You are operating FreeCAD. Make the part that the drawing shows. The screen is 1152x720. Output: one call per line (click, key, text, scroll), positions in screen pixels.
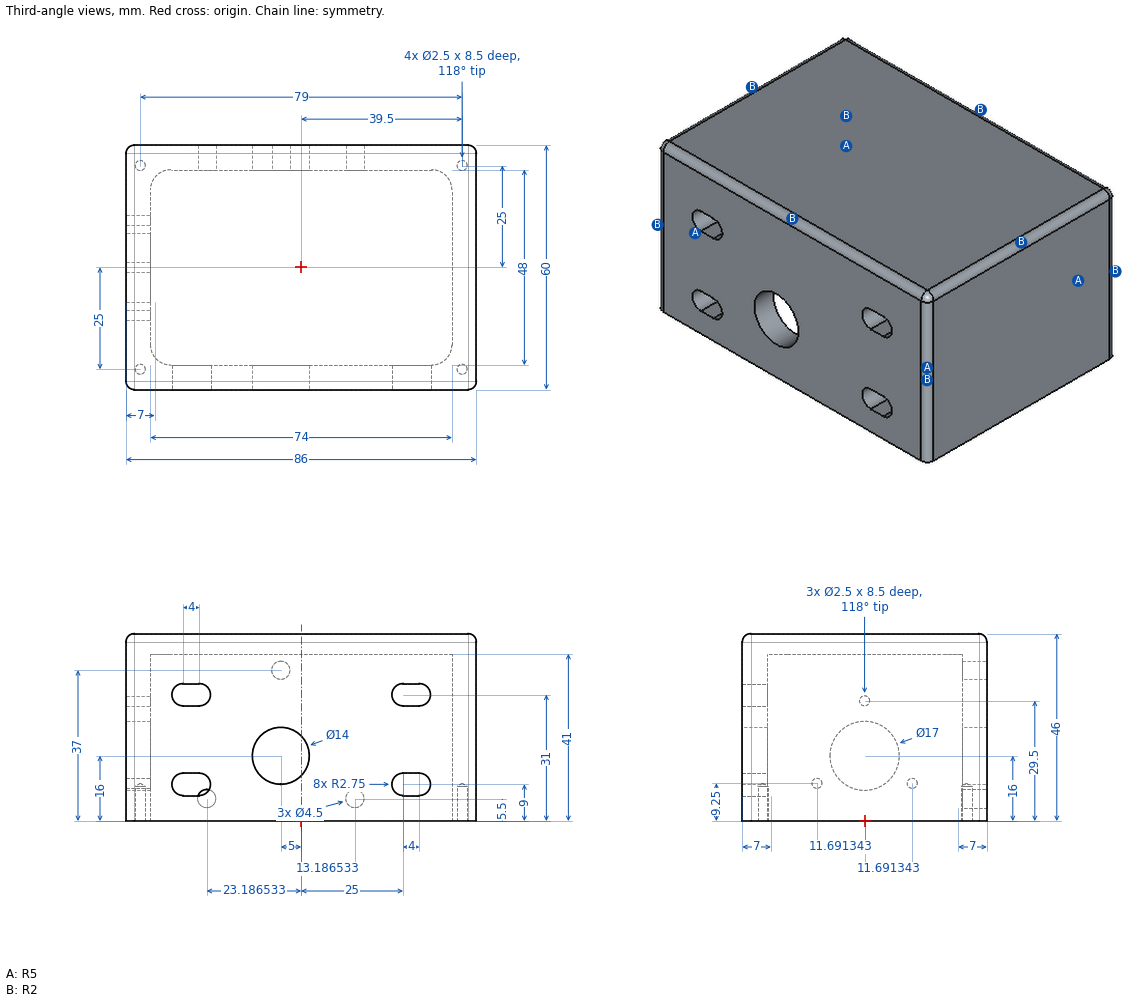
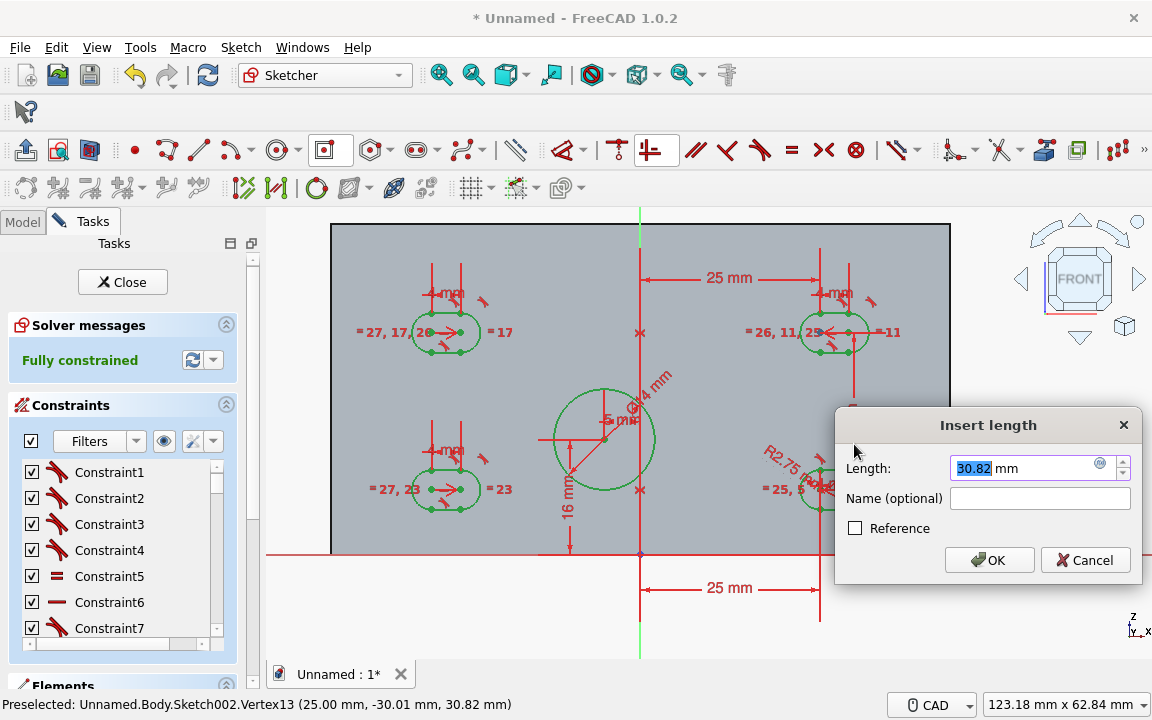
text(31)
key(Return)
key(Escape)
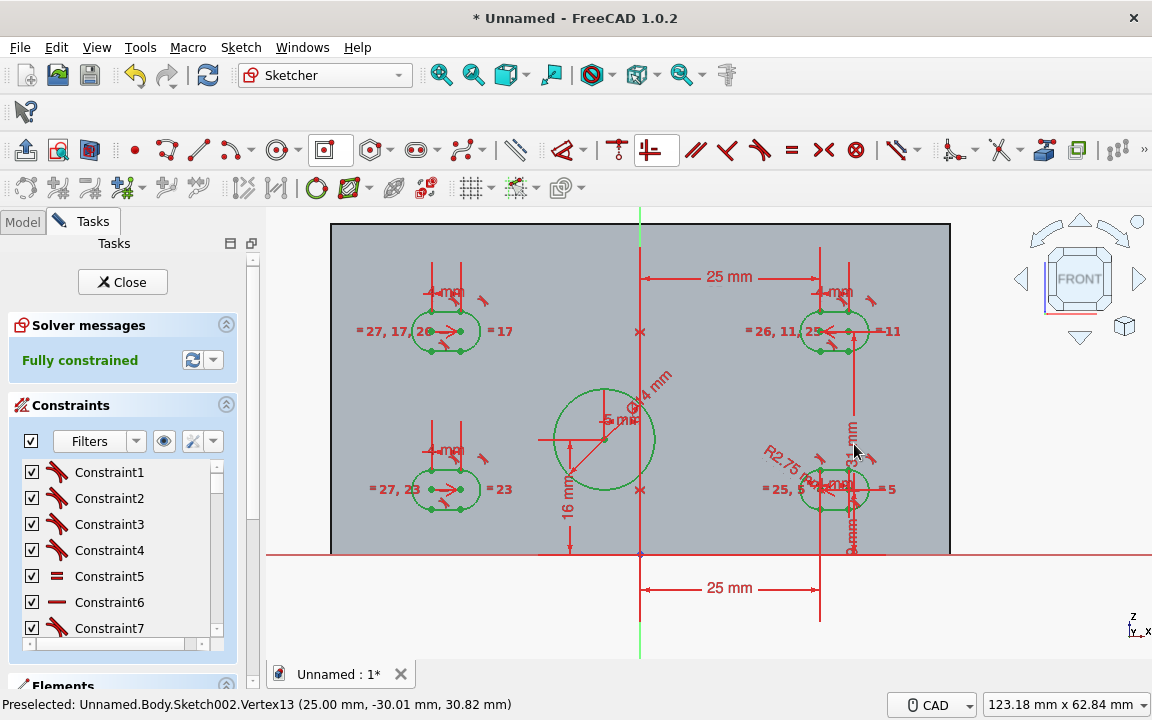
click(123, 282)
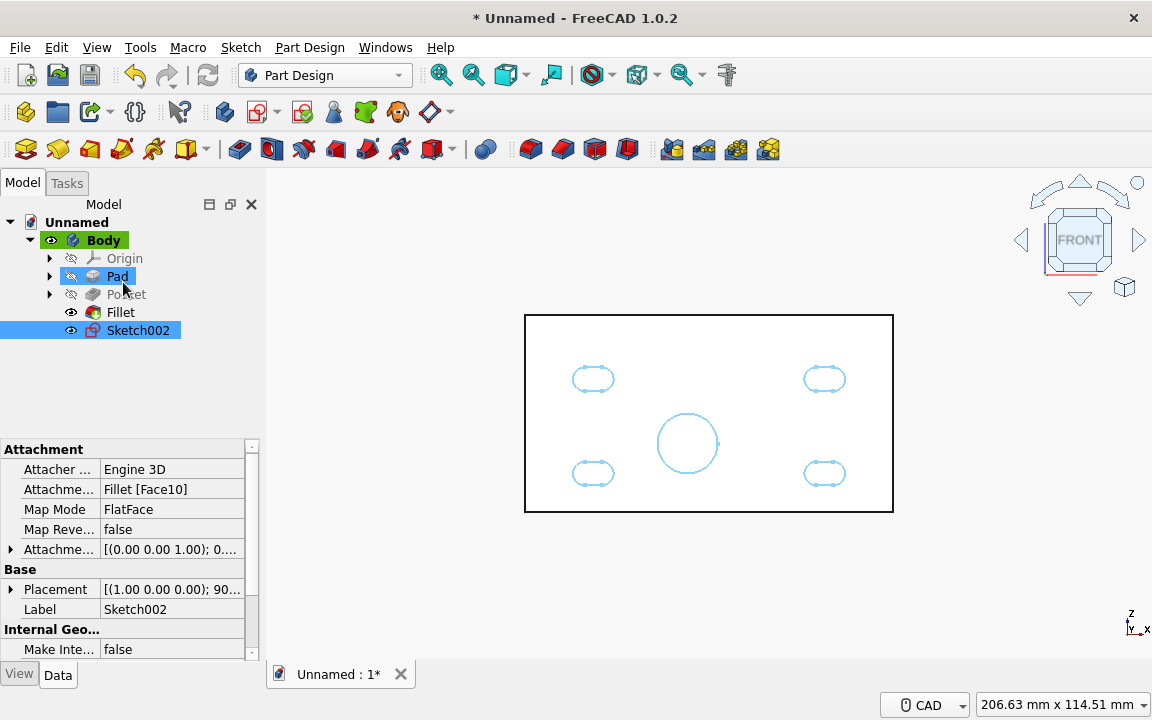
click(240, 150)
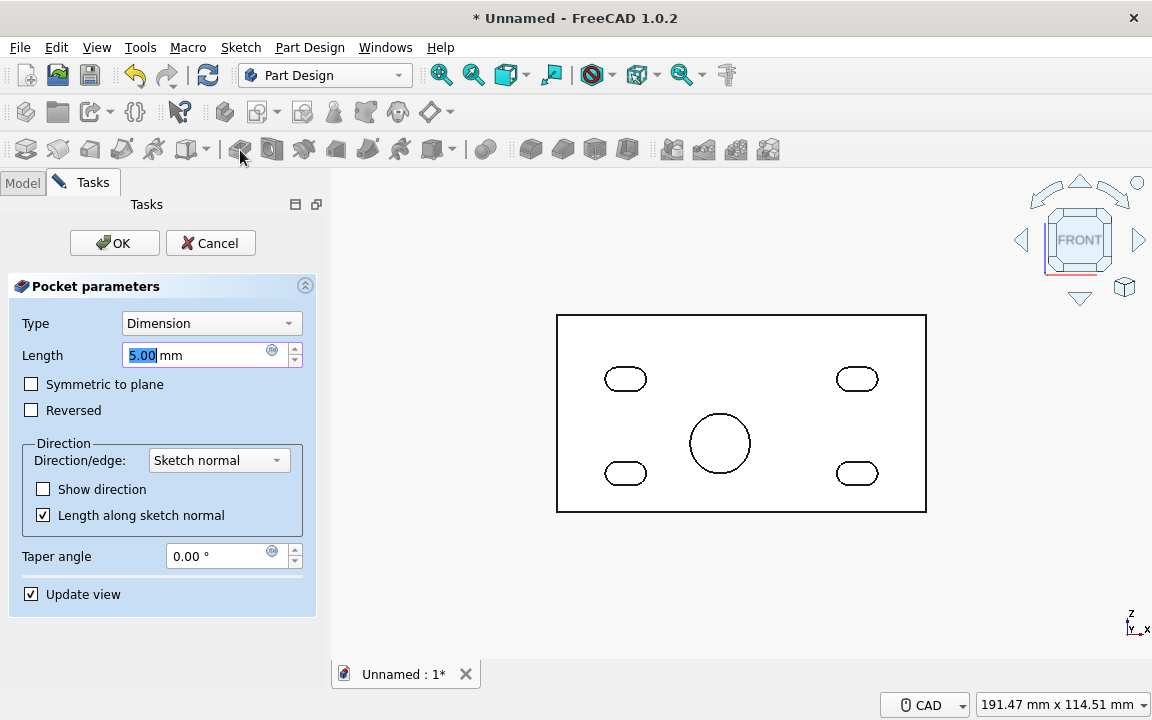
text(7)
key(Tab)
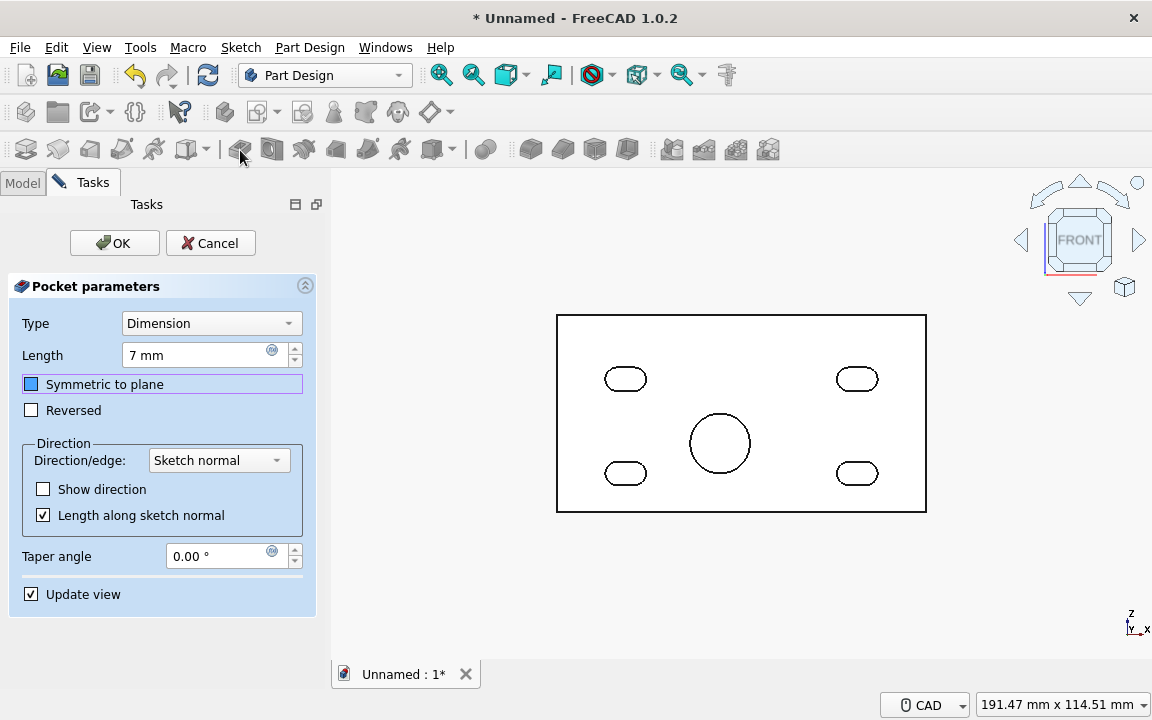
click(115, 243)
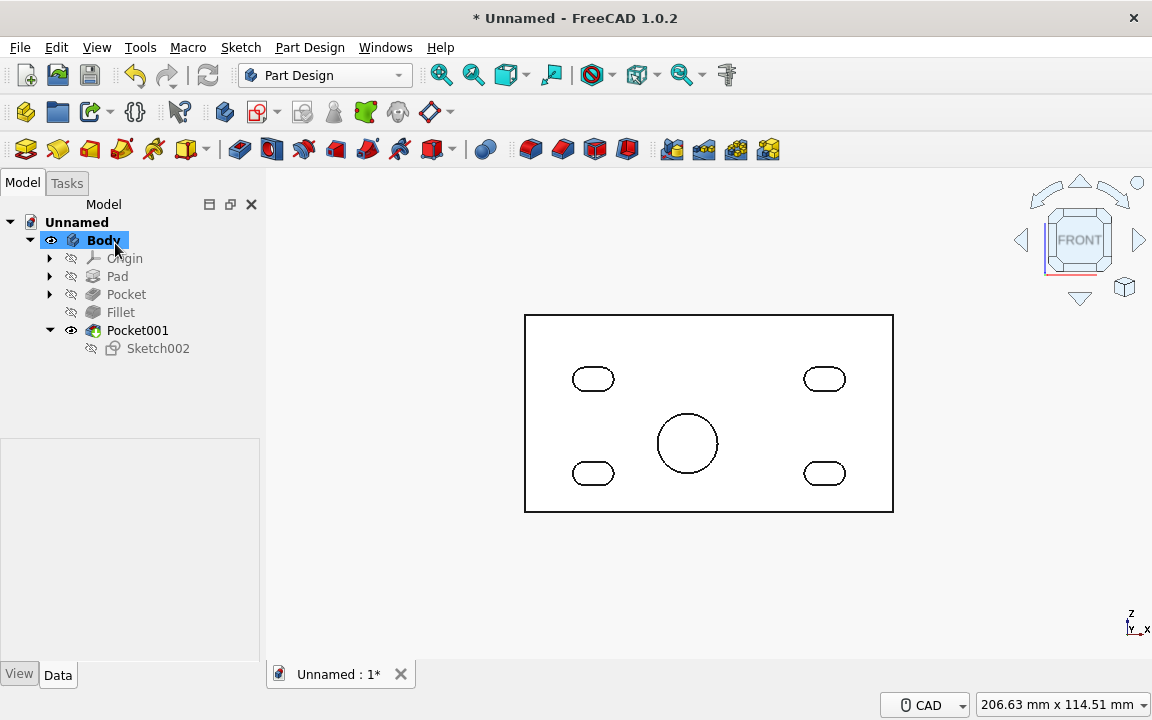
key(v)
key(f)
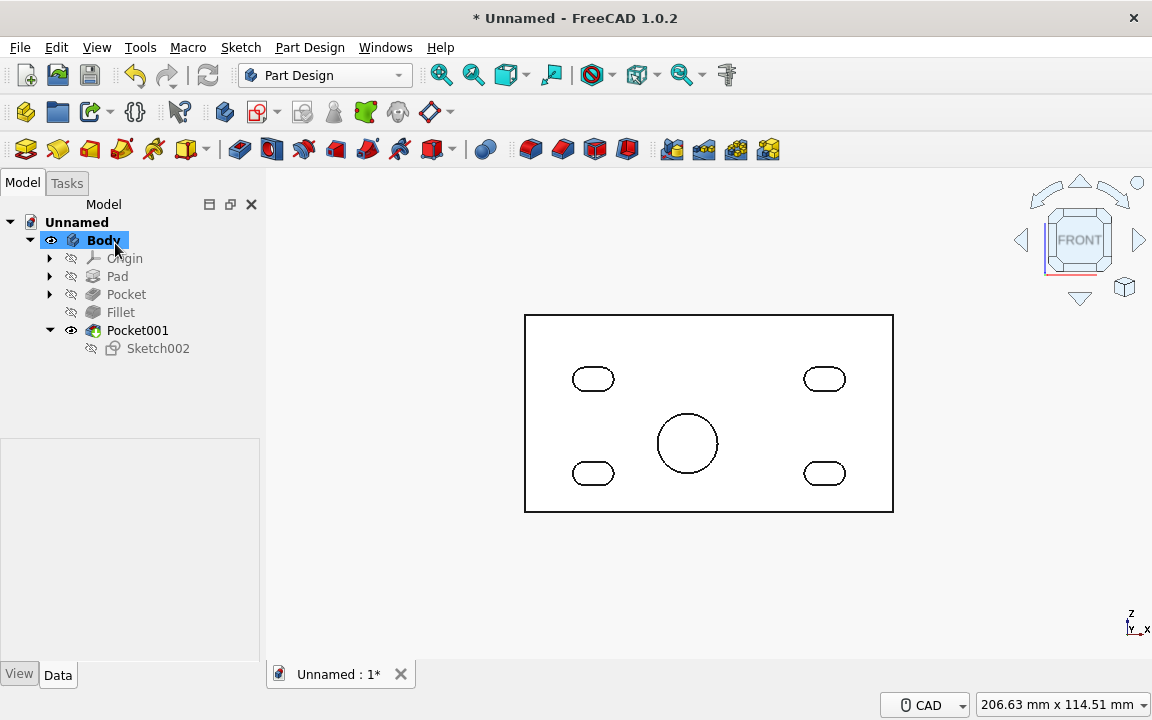
click(50, 258)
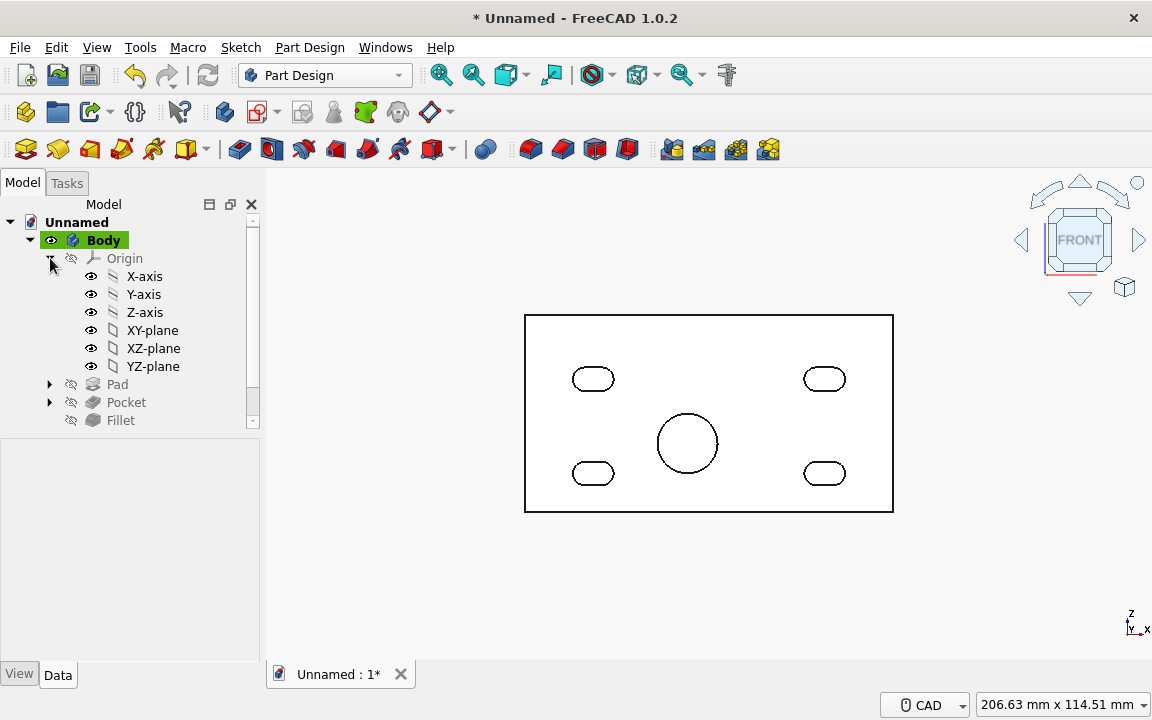
click(136, 348)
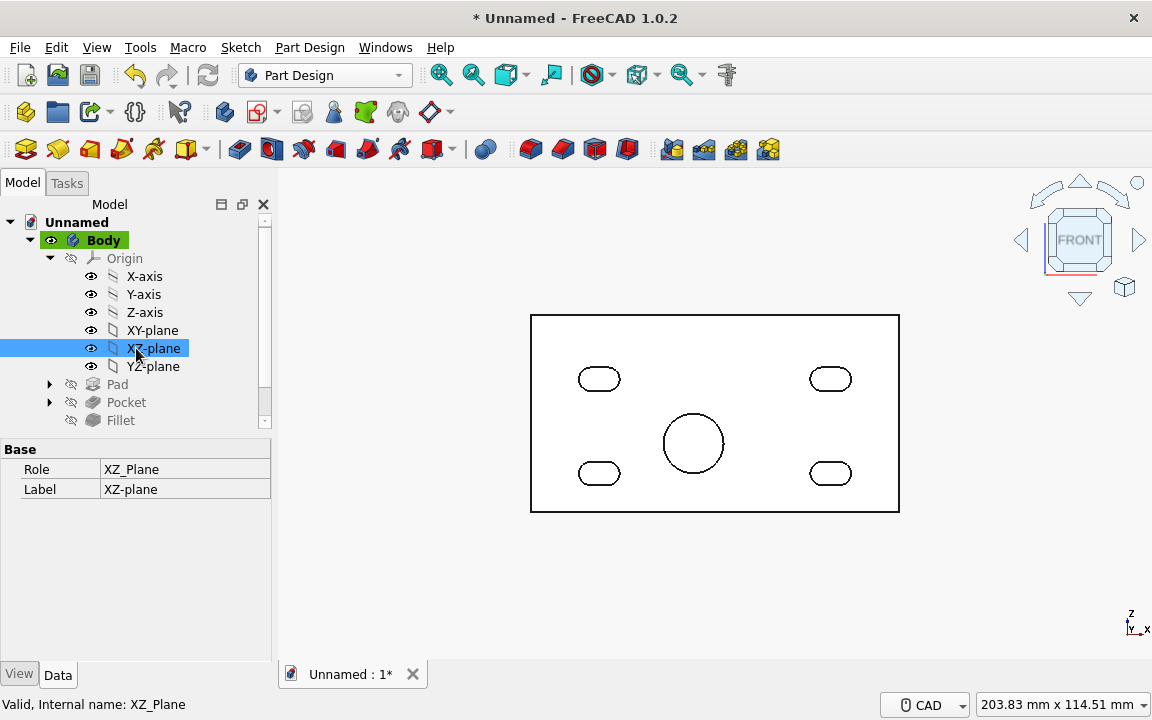
click(430, 112)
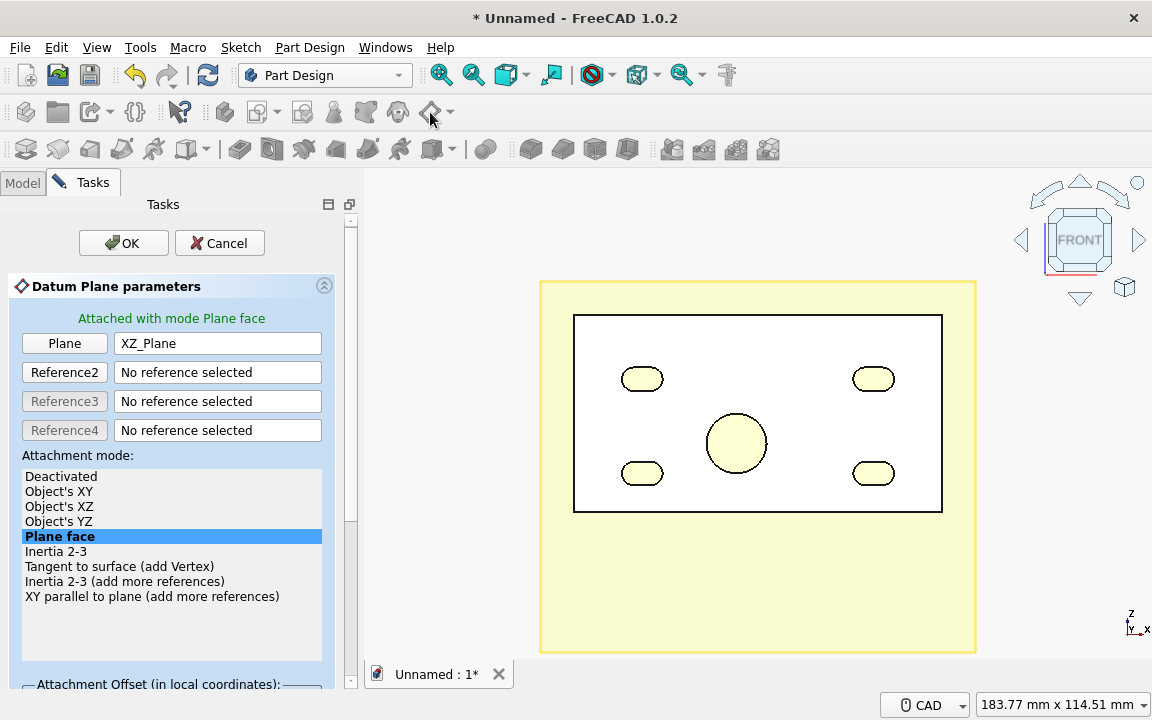
scroll(351, 451, down, 3)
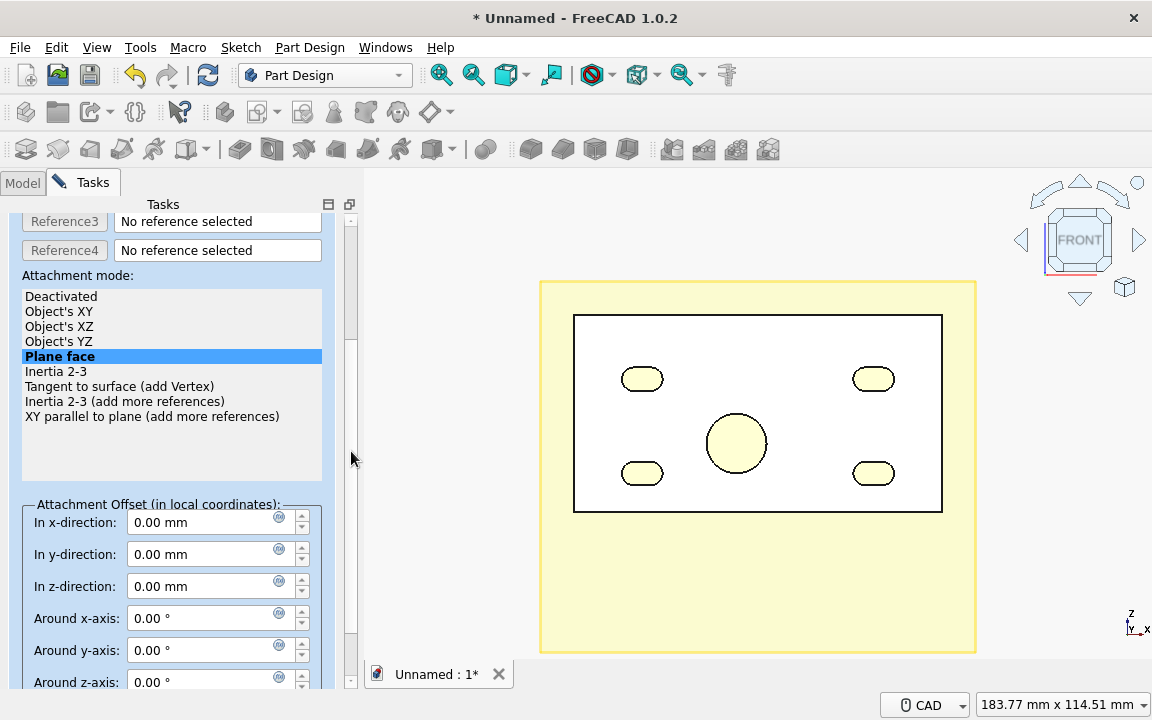
triple_click(210, 586)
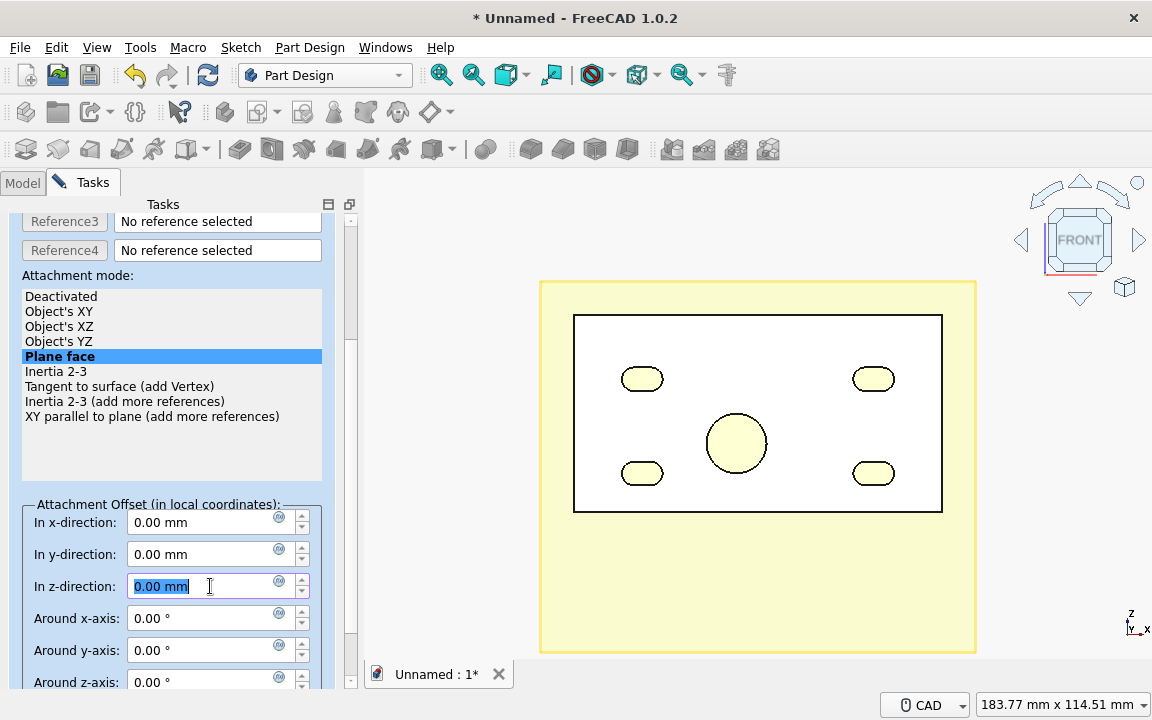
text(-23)
key(Tab)